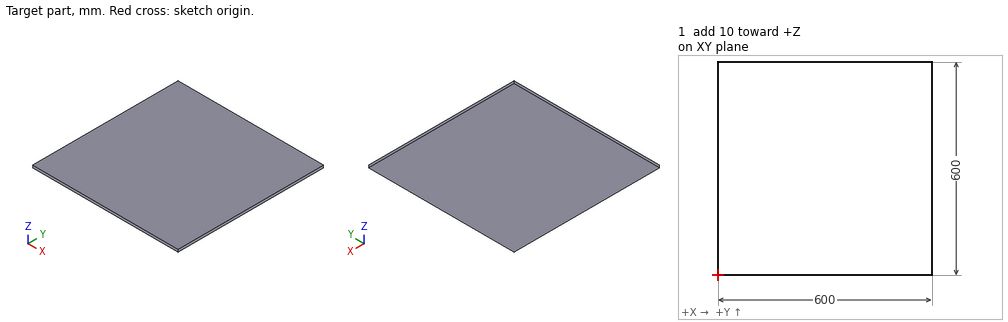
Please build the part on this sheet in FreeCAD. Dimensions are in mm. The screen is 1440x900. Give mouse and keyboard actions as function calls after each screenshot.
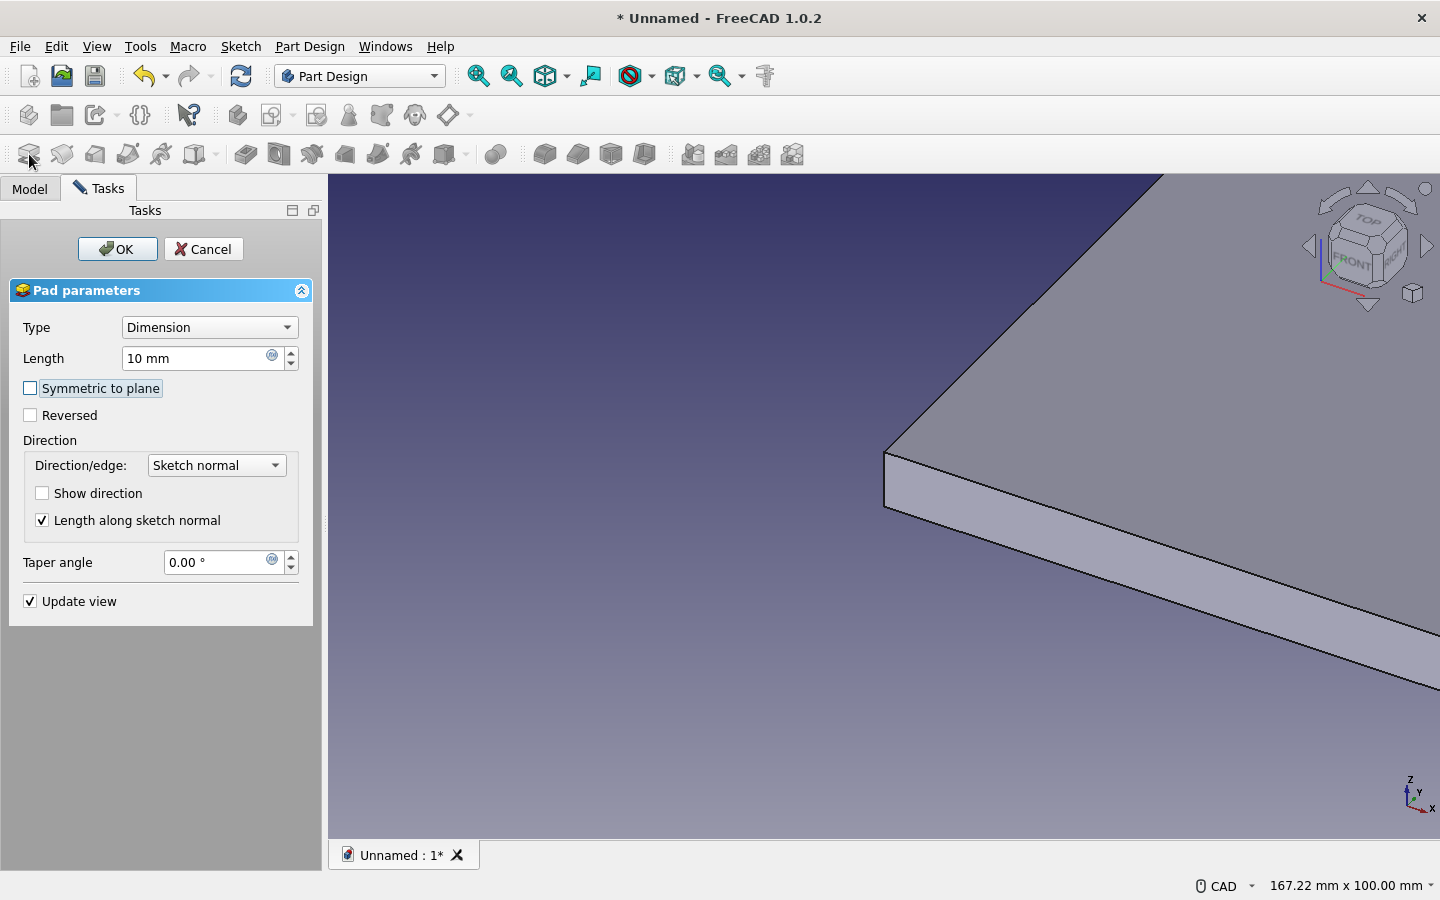
click(118, 249)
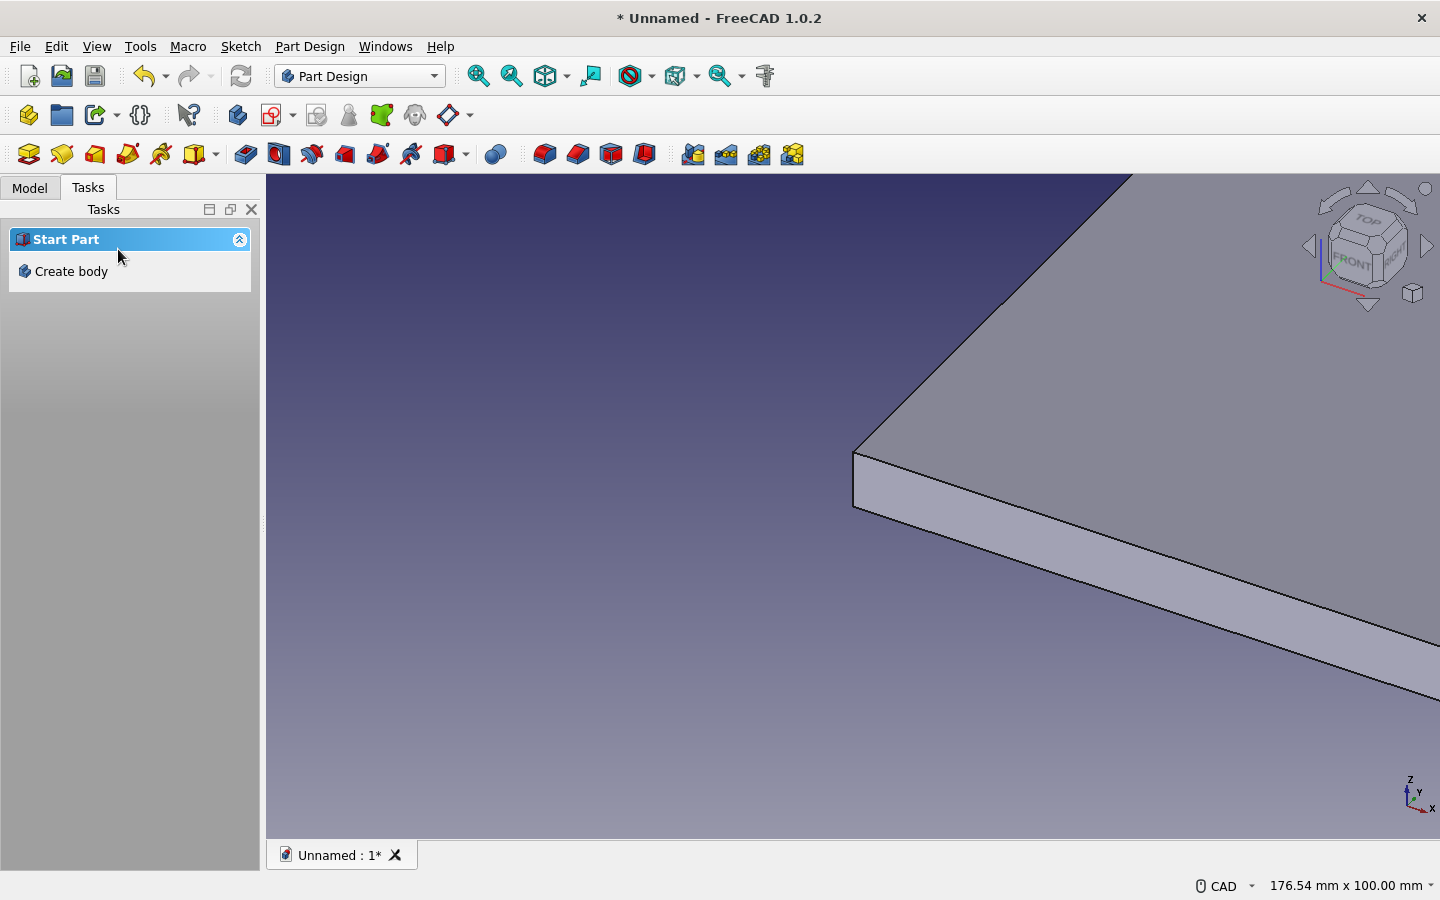
key(0)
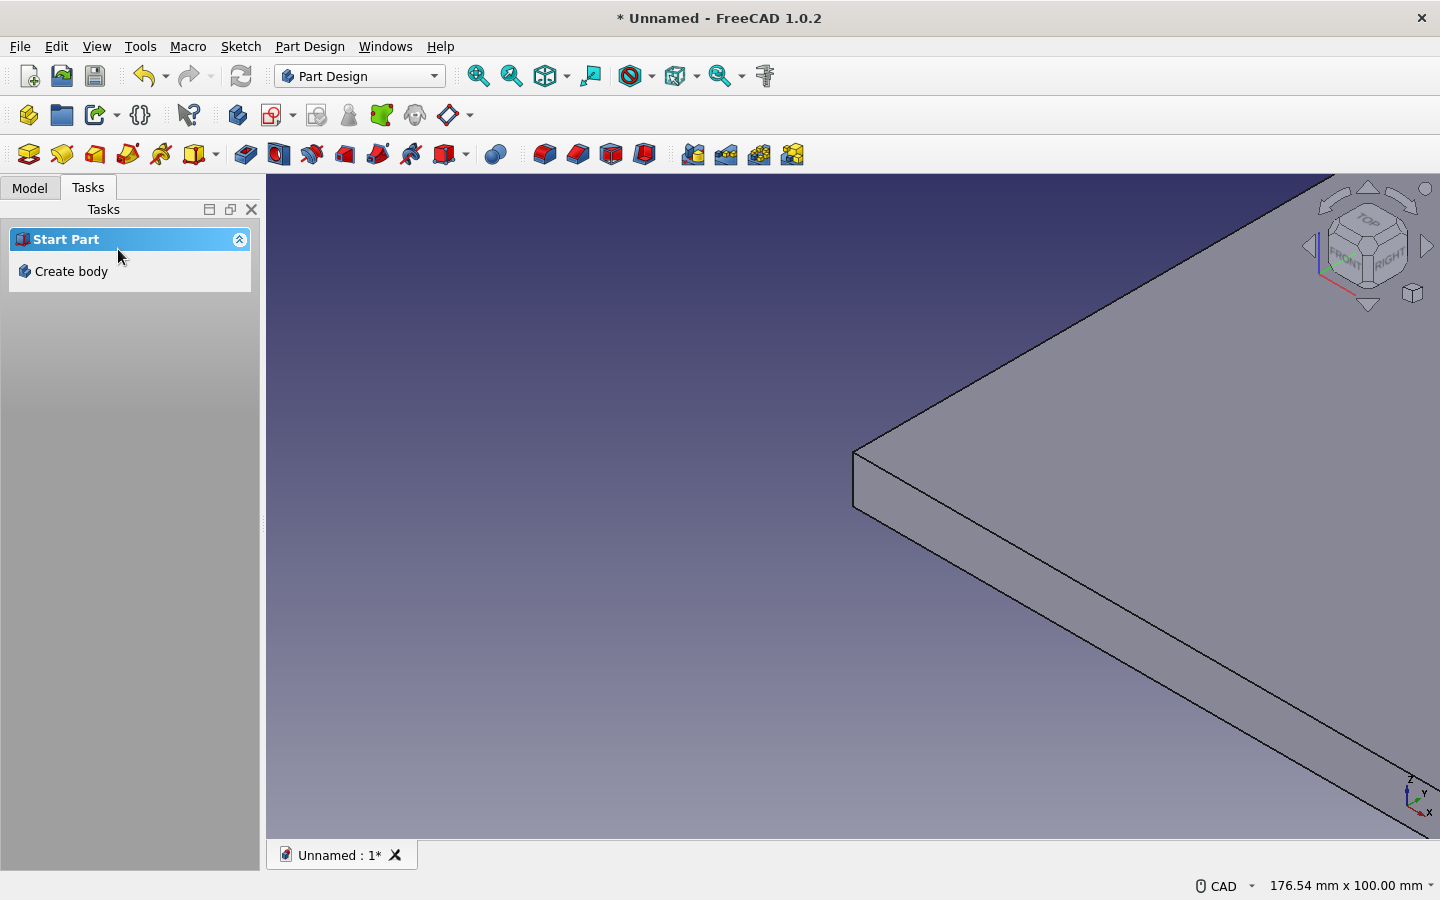
click(479, 76)